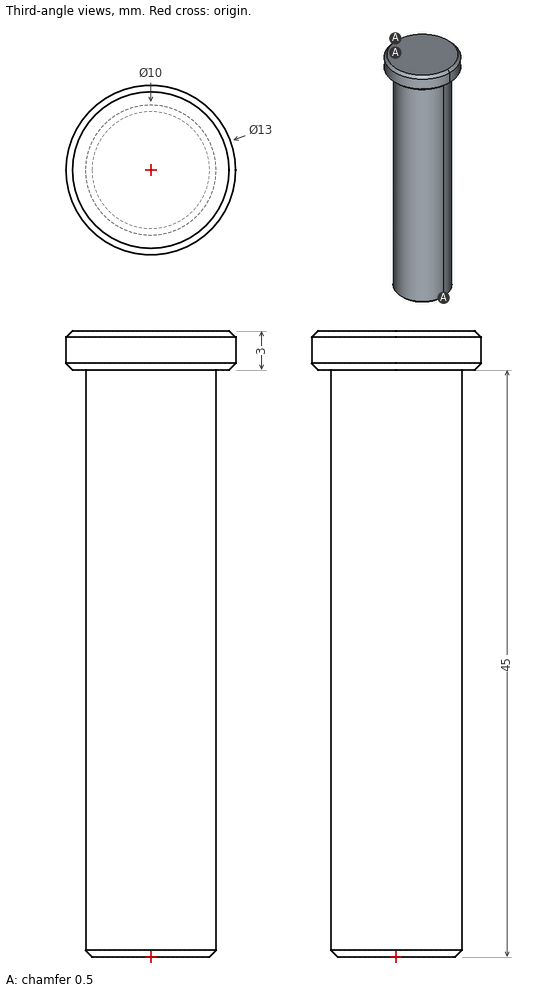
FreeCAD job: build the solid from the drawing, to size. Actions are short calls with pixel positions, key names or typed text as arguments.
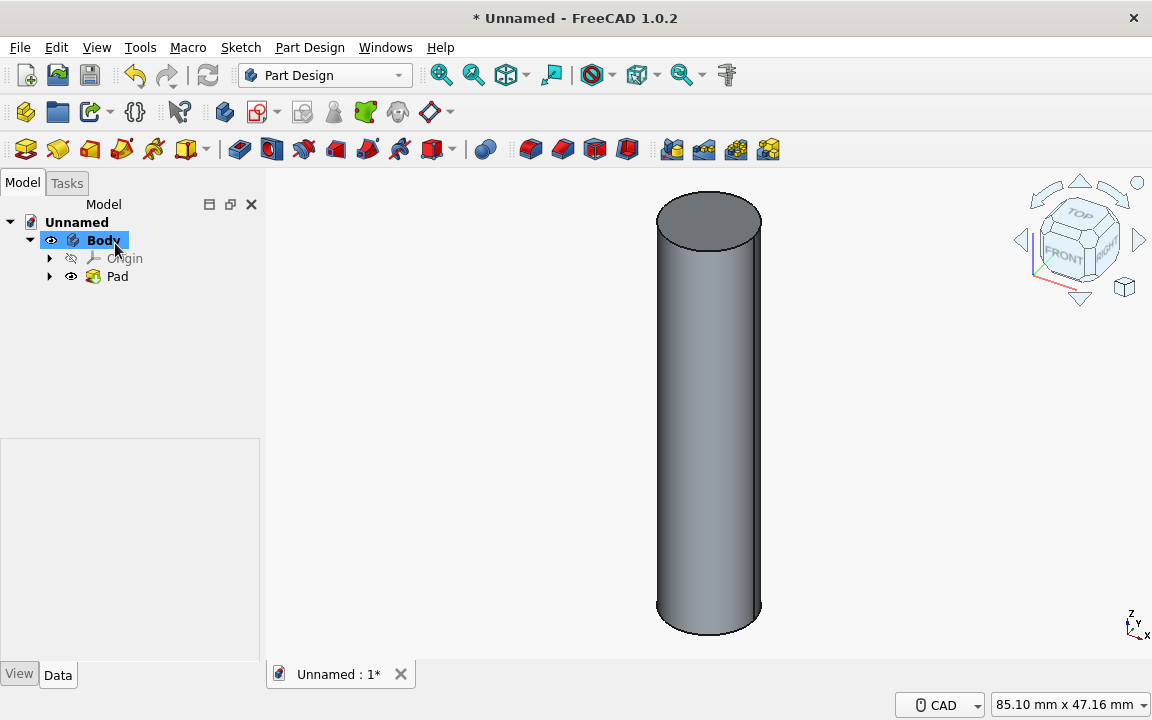
click(709, 221)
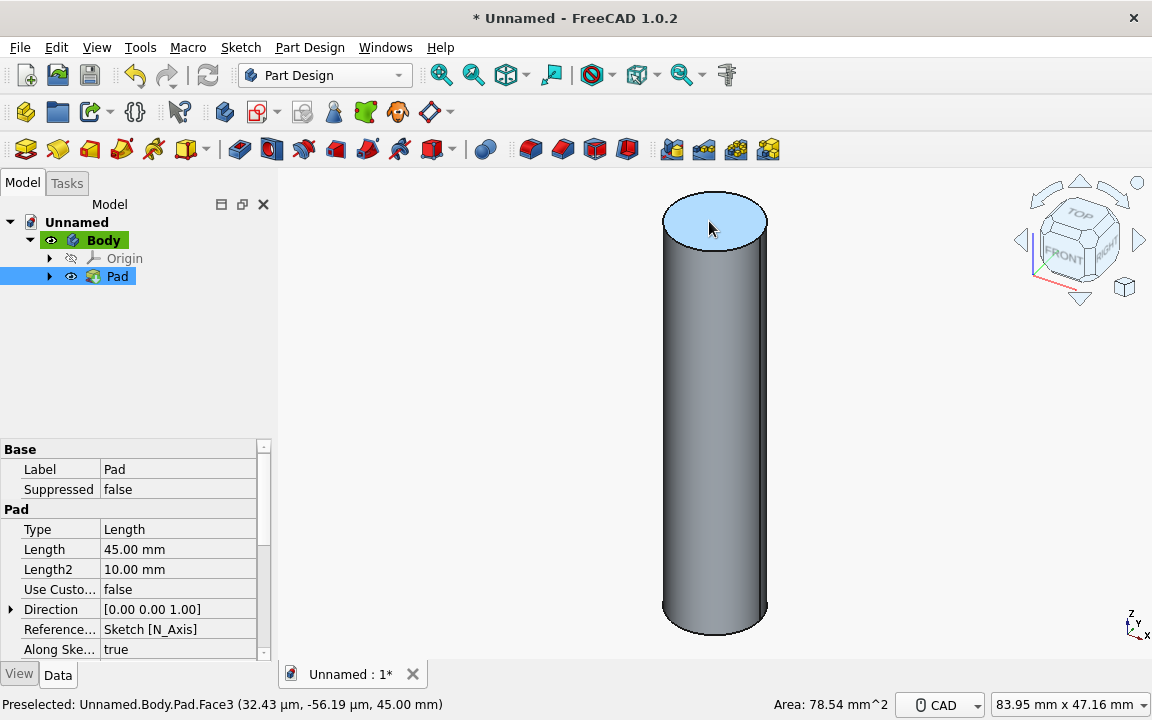
click(258, 112)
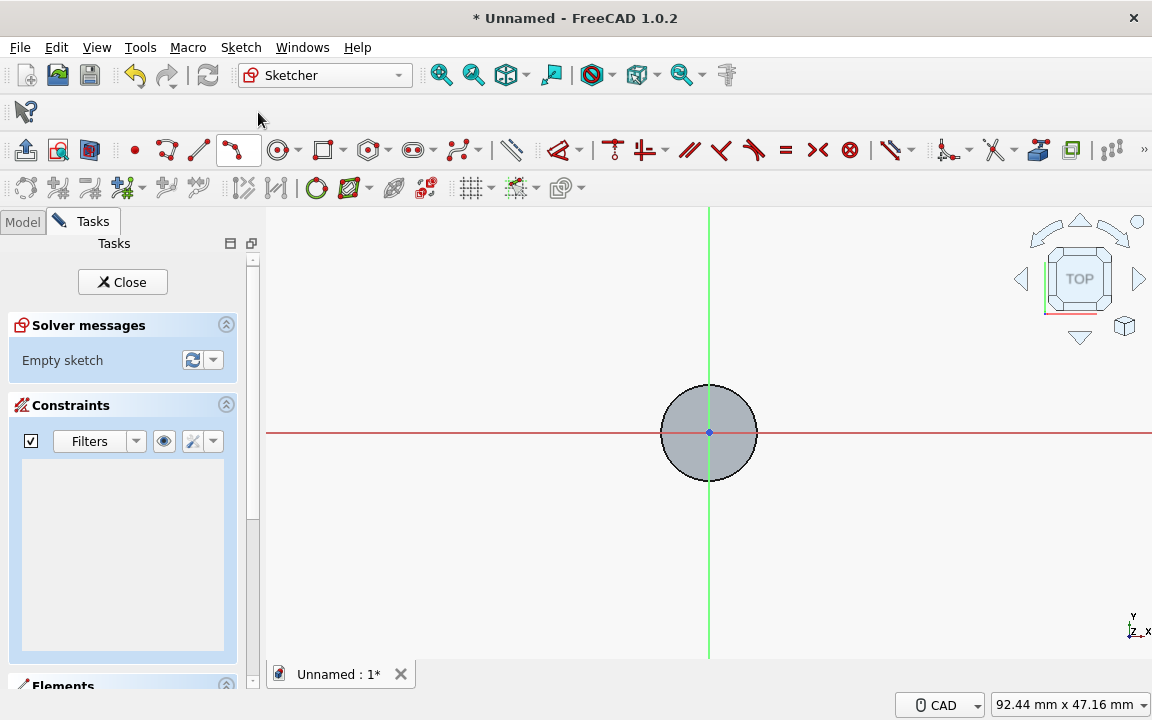
scroll(765, 433, up, 4)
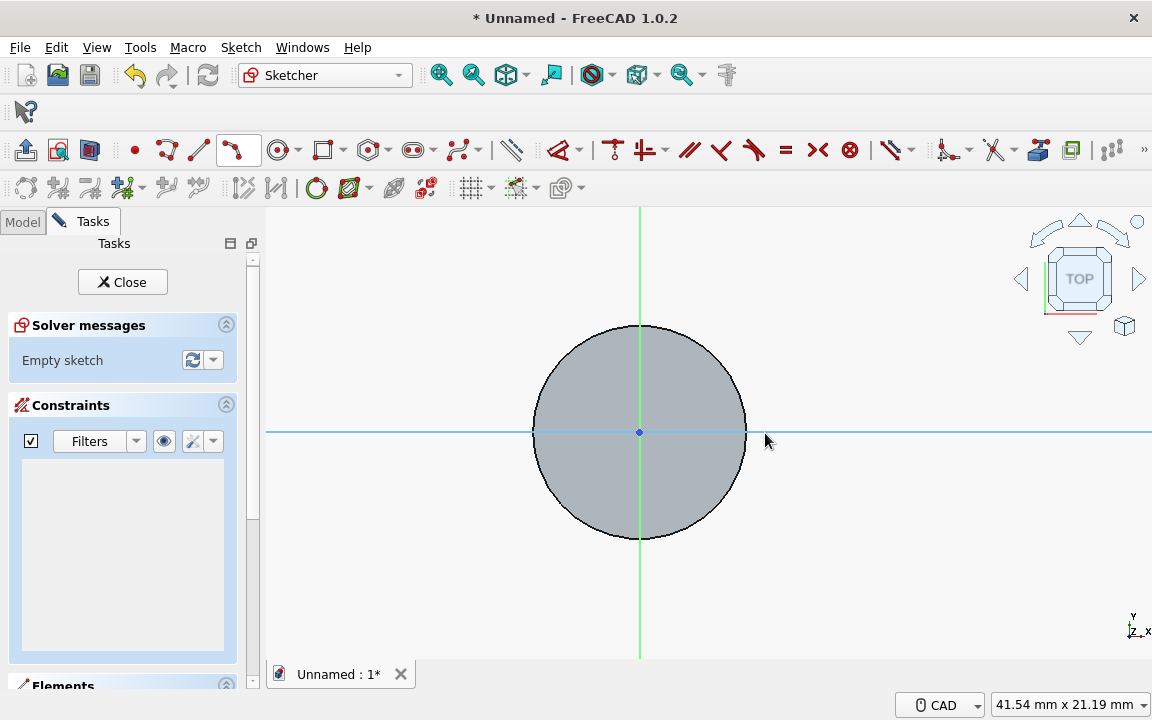
key(g)
key(c)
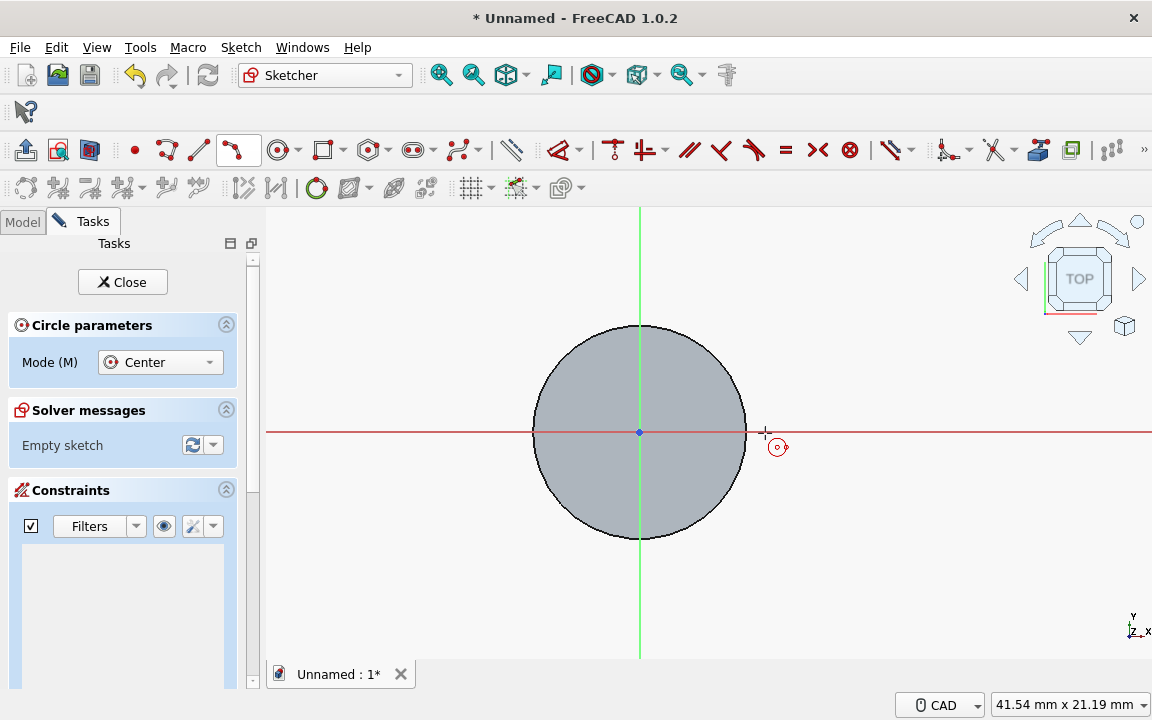
click(640, 432)
move(738, 334)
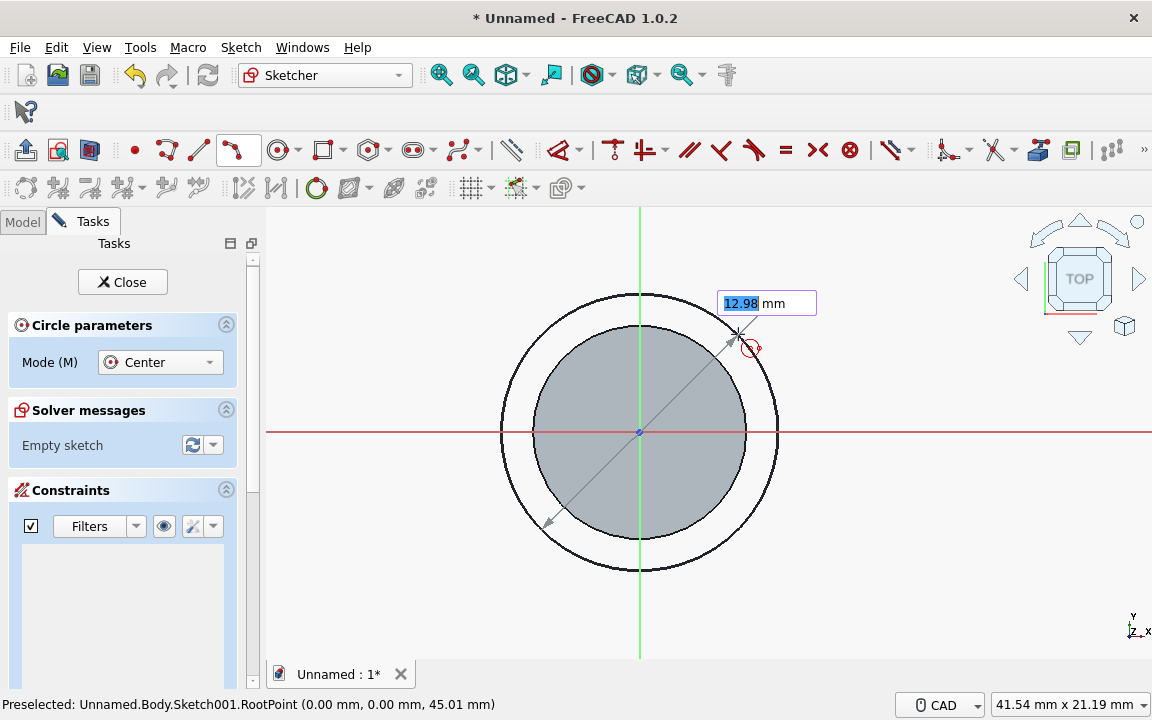
text(13)
key(Return)
key(Escape)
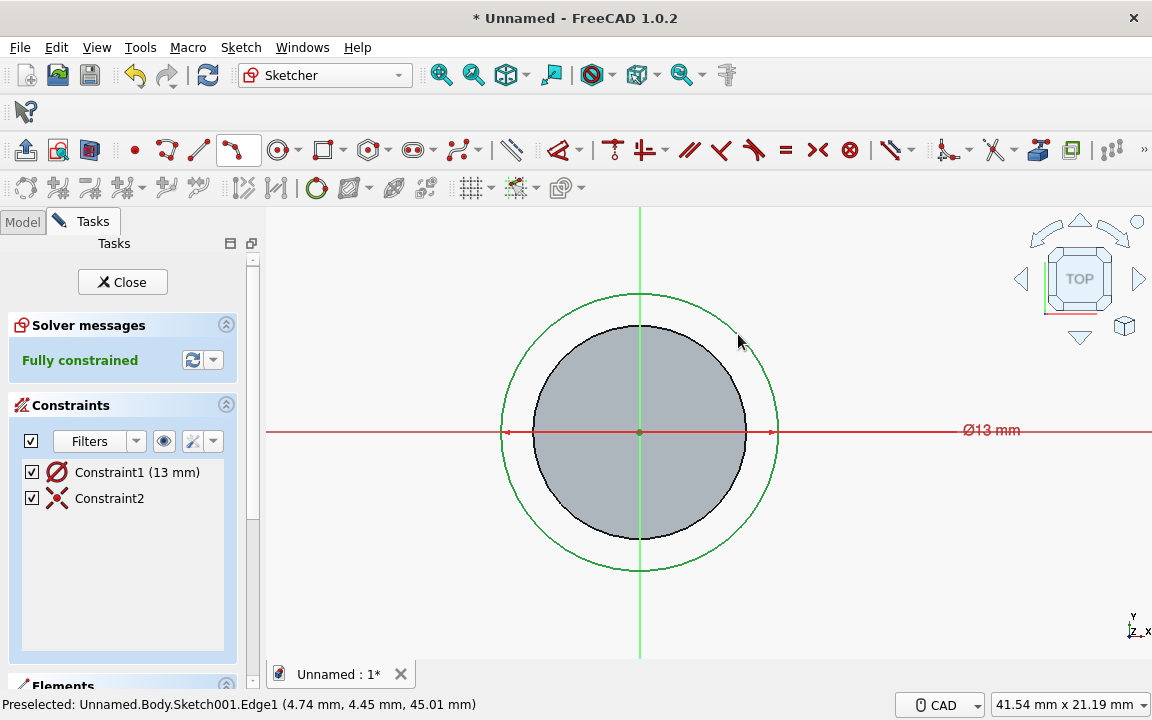
click(123, 282)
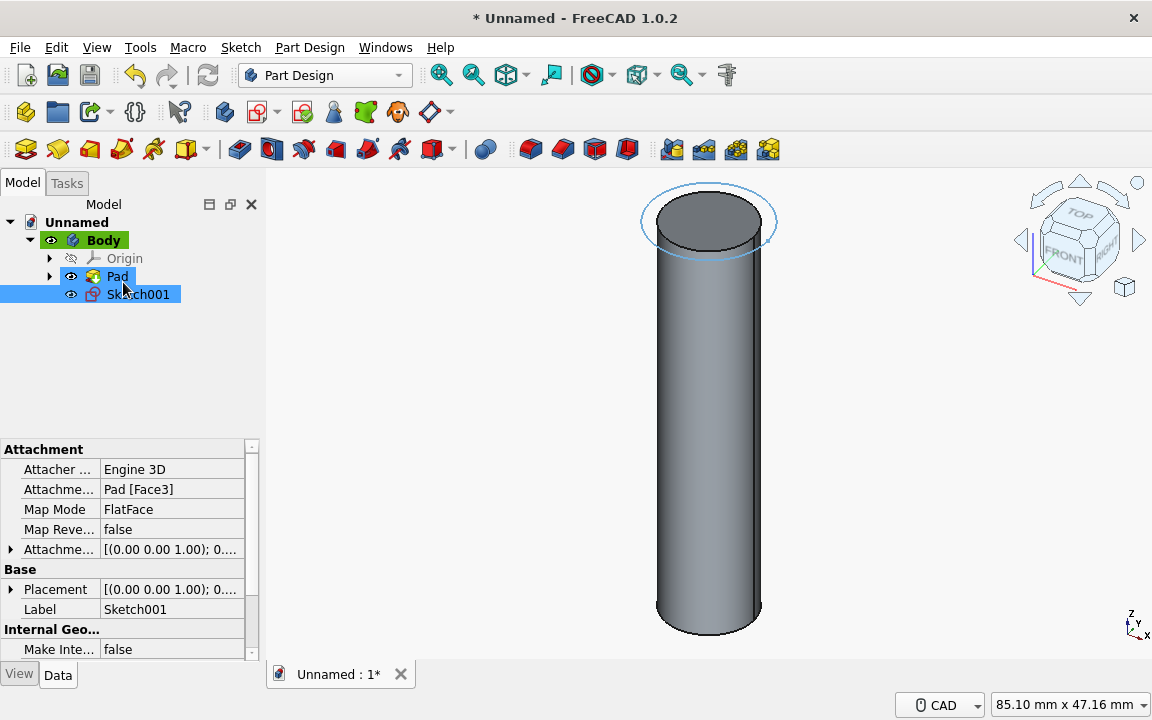
click(26, 150)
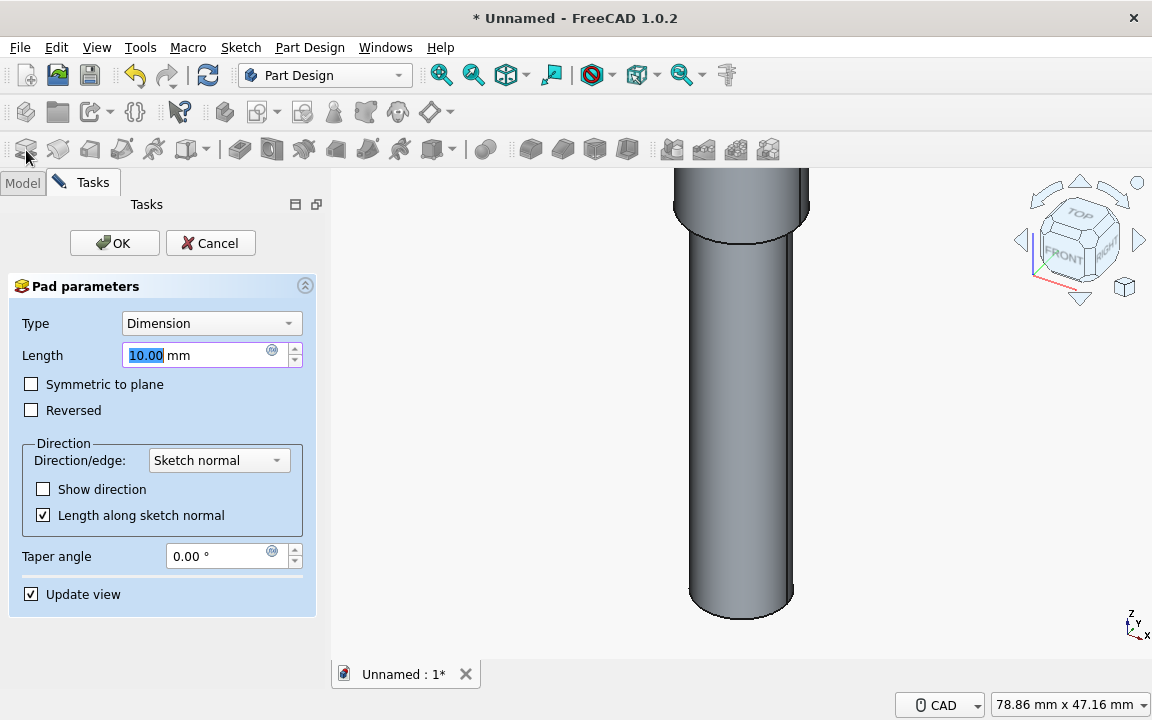
text(3)
key(Tab)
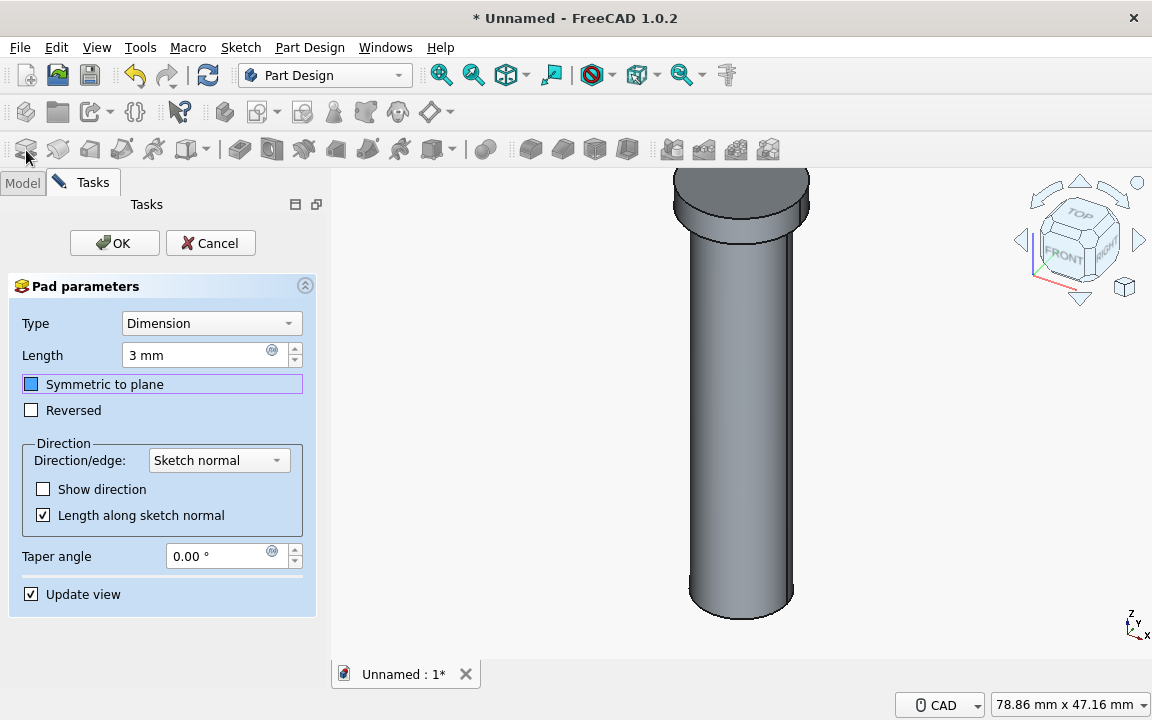
click(115, 243)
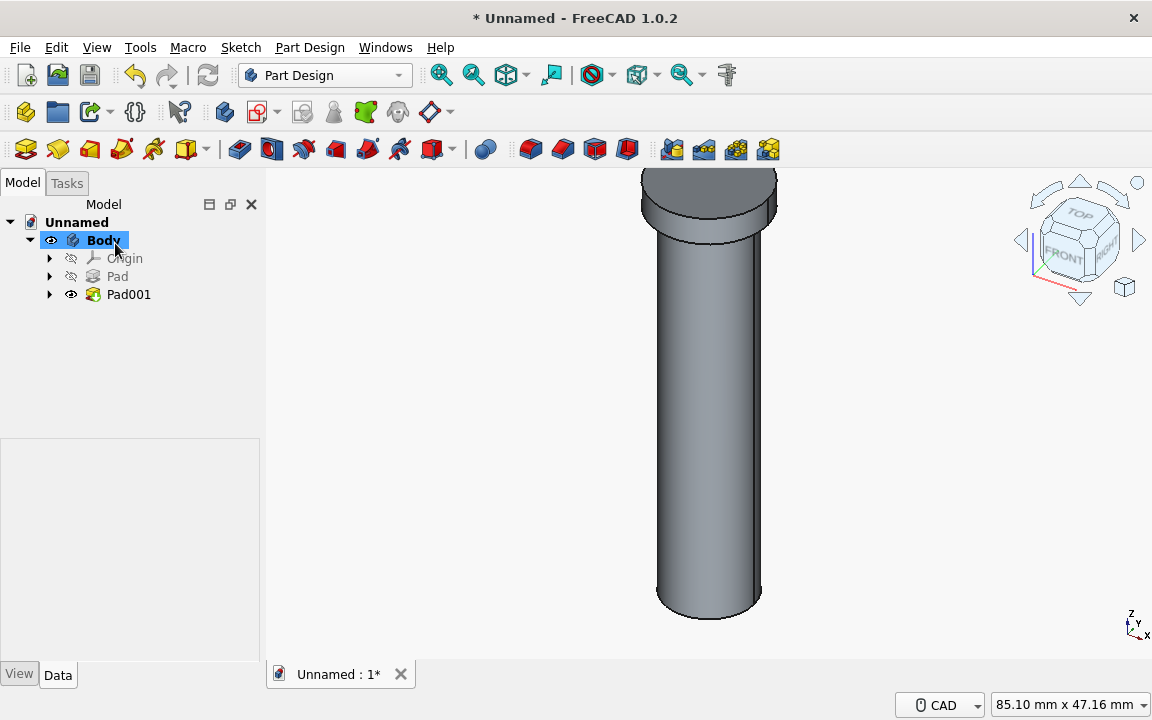
click(442, 76)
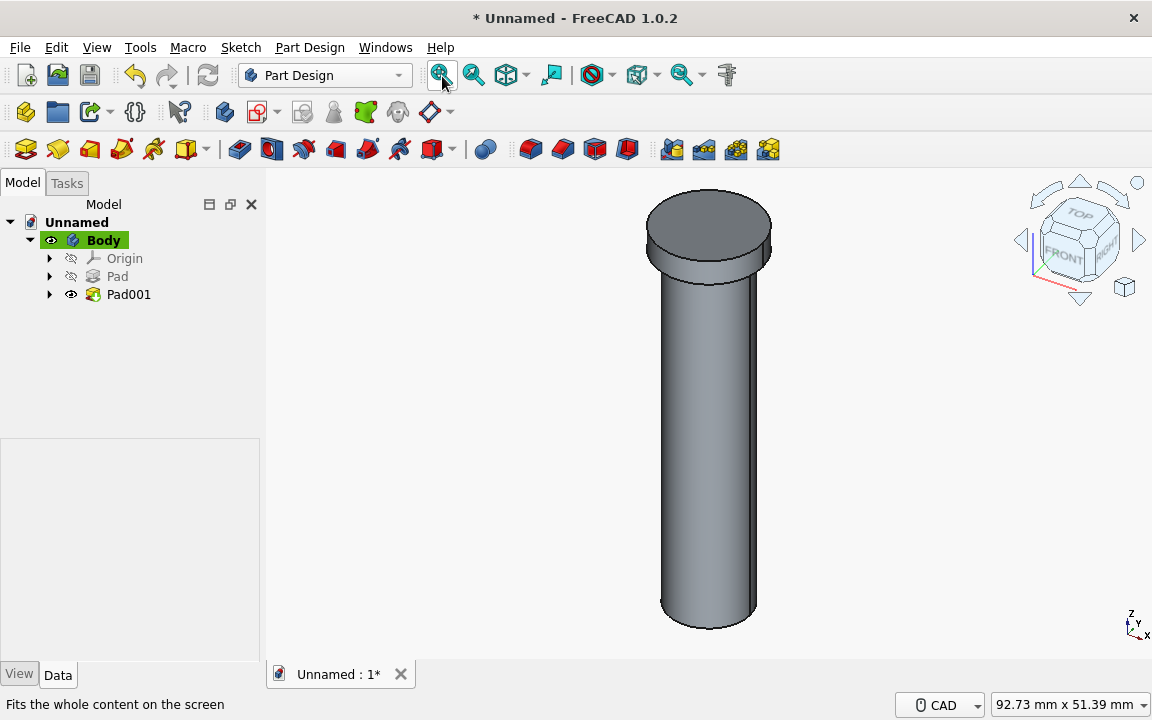
click(673, 619)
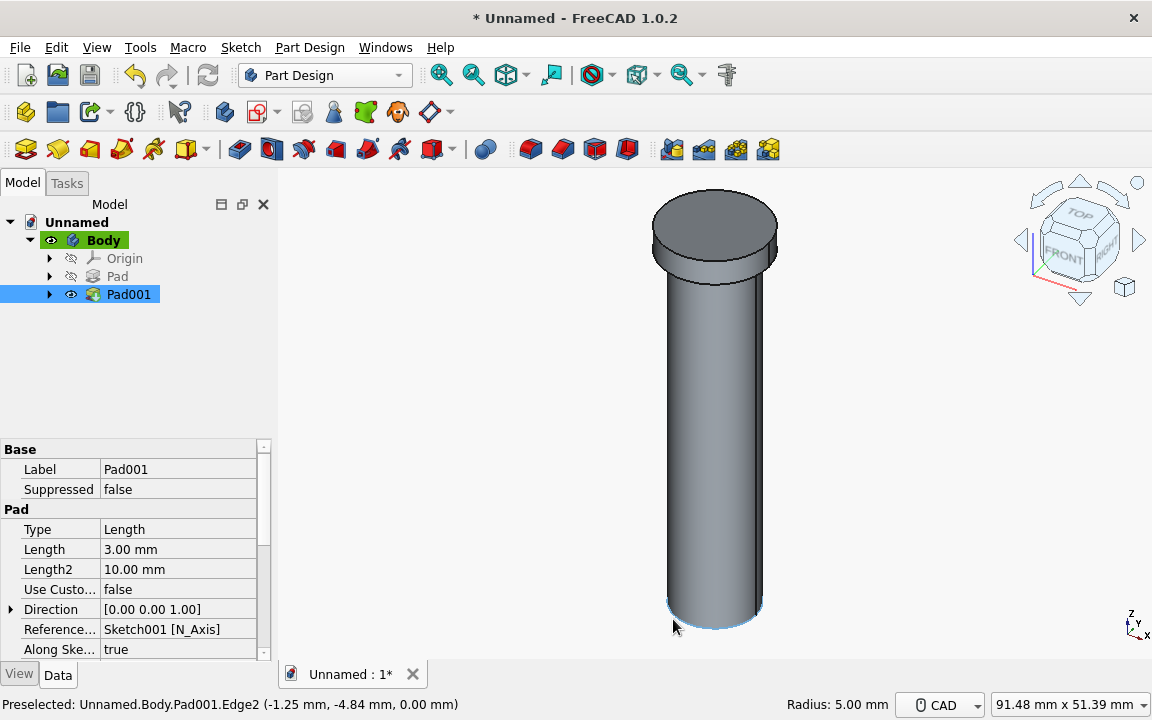
click(653, 228, ctrl)